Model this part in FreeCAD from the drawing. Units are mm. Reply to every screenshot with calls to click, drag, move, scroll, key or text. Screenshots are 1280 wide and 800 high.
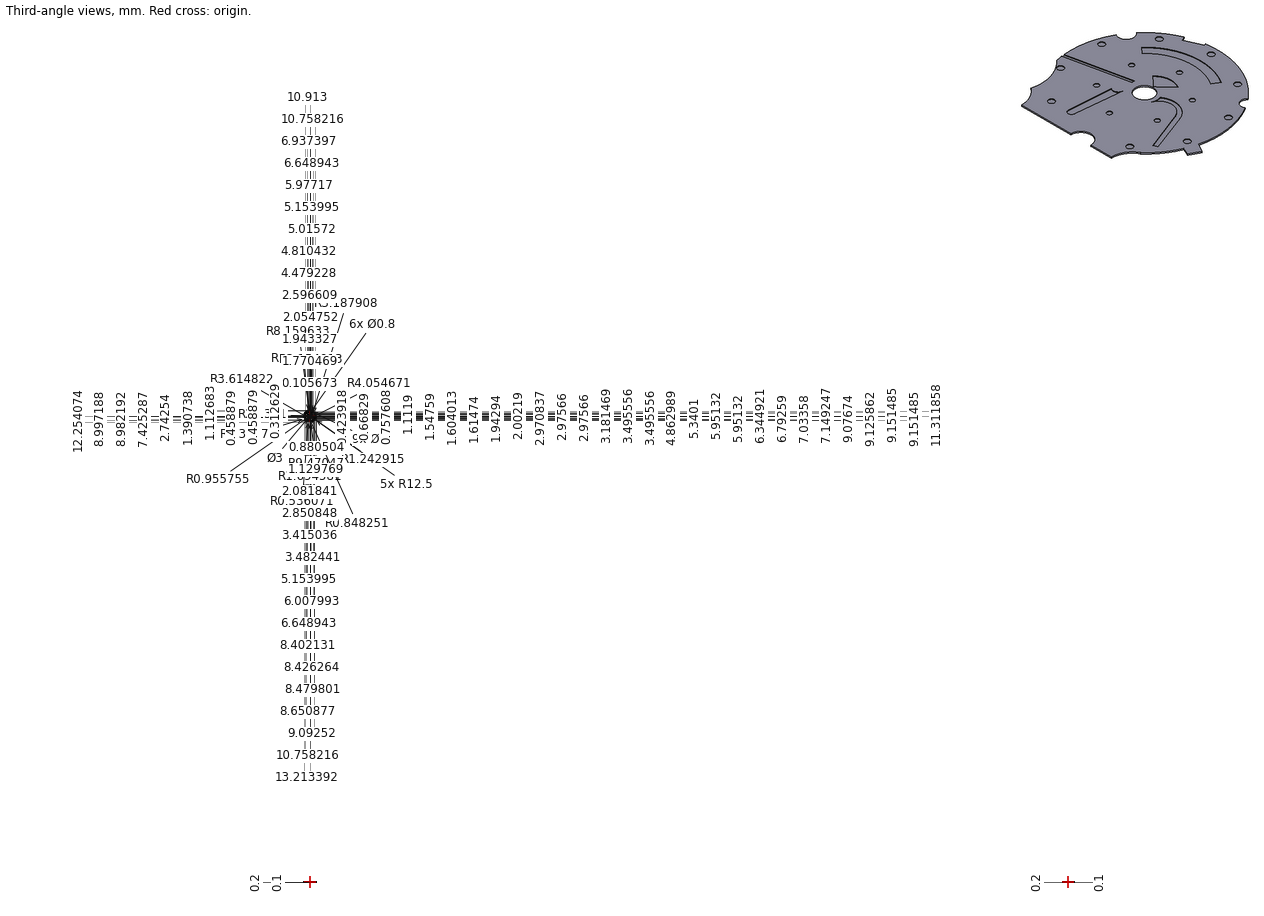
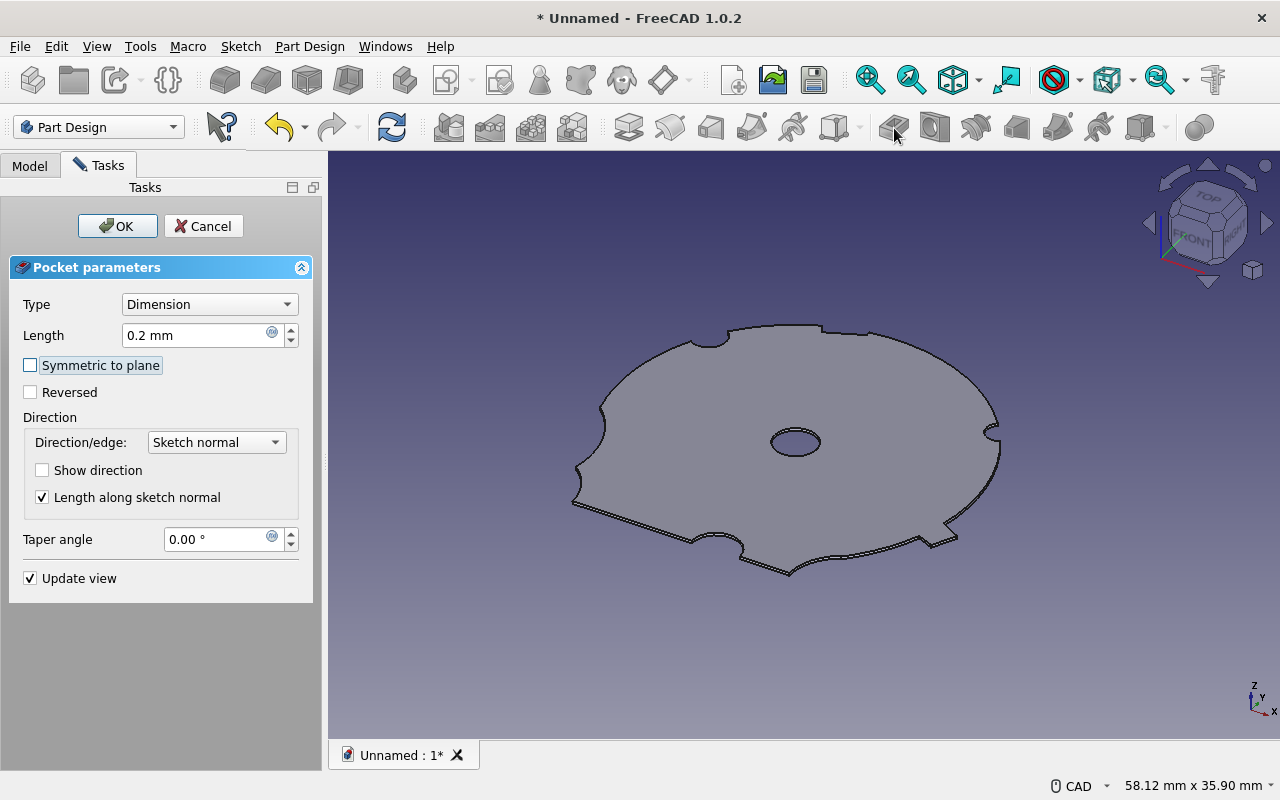
click(118, 226)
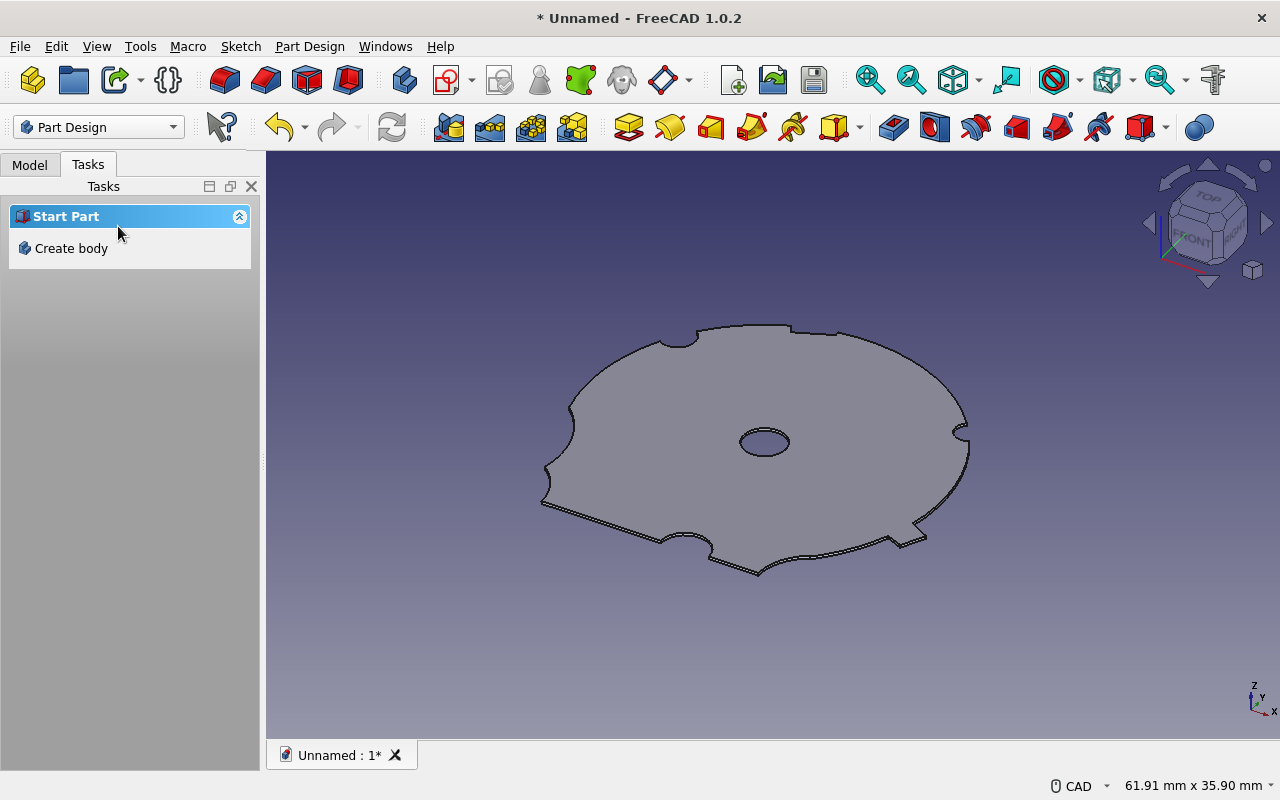
click(668, 408)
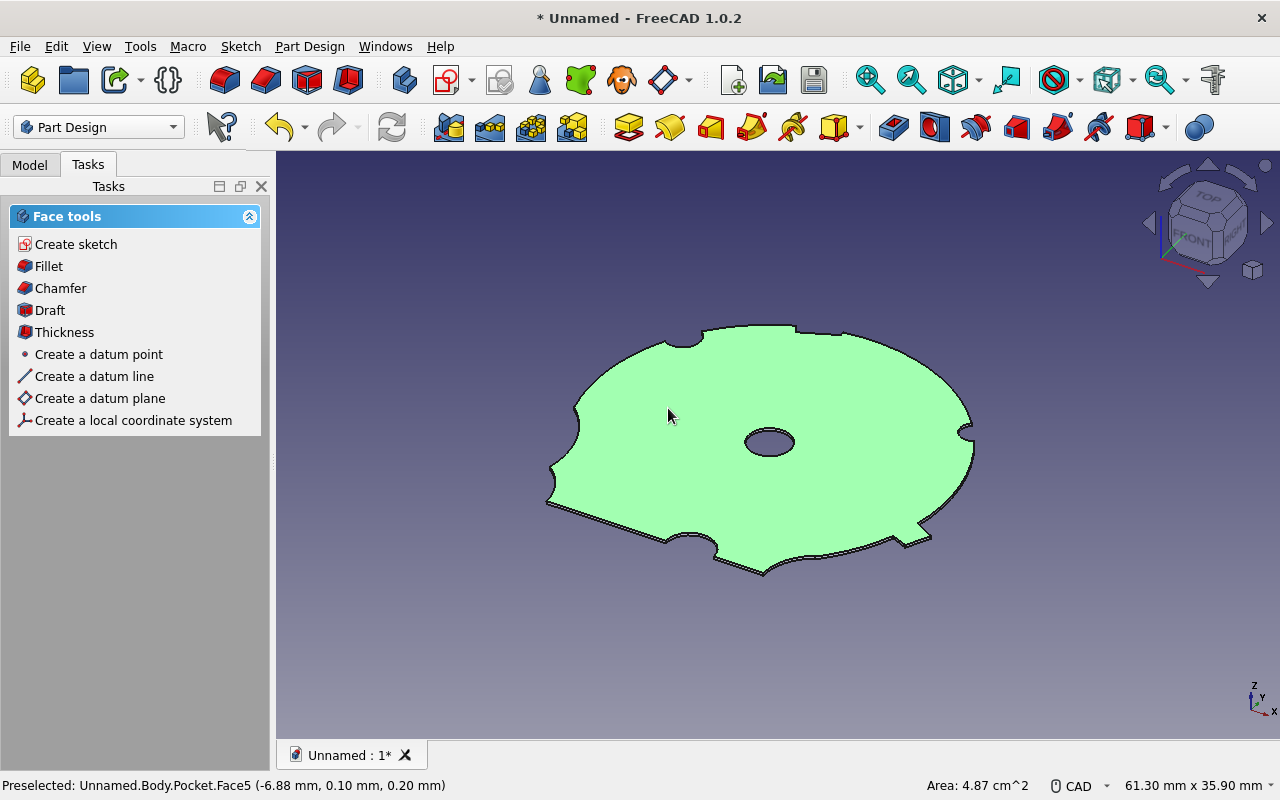
click(446, 80)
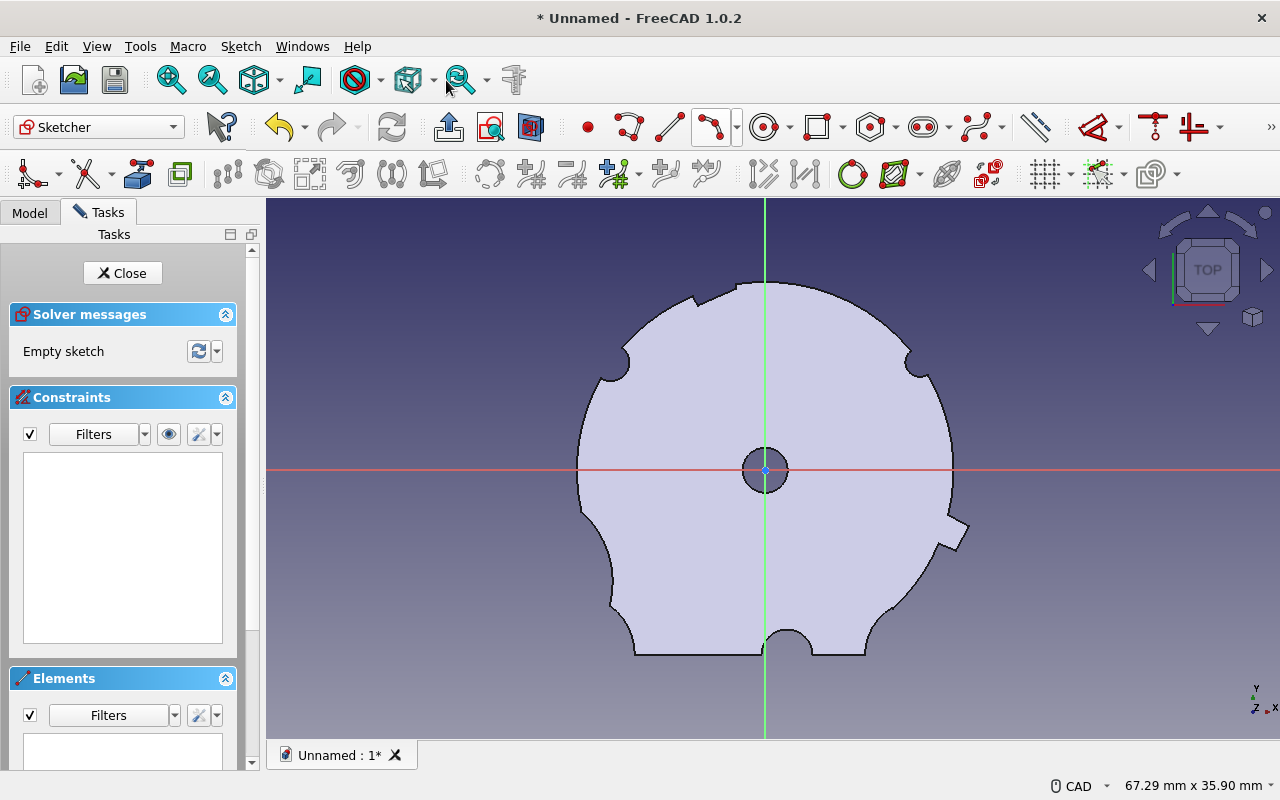
key(g)
key(c)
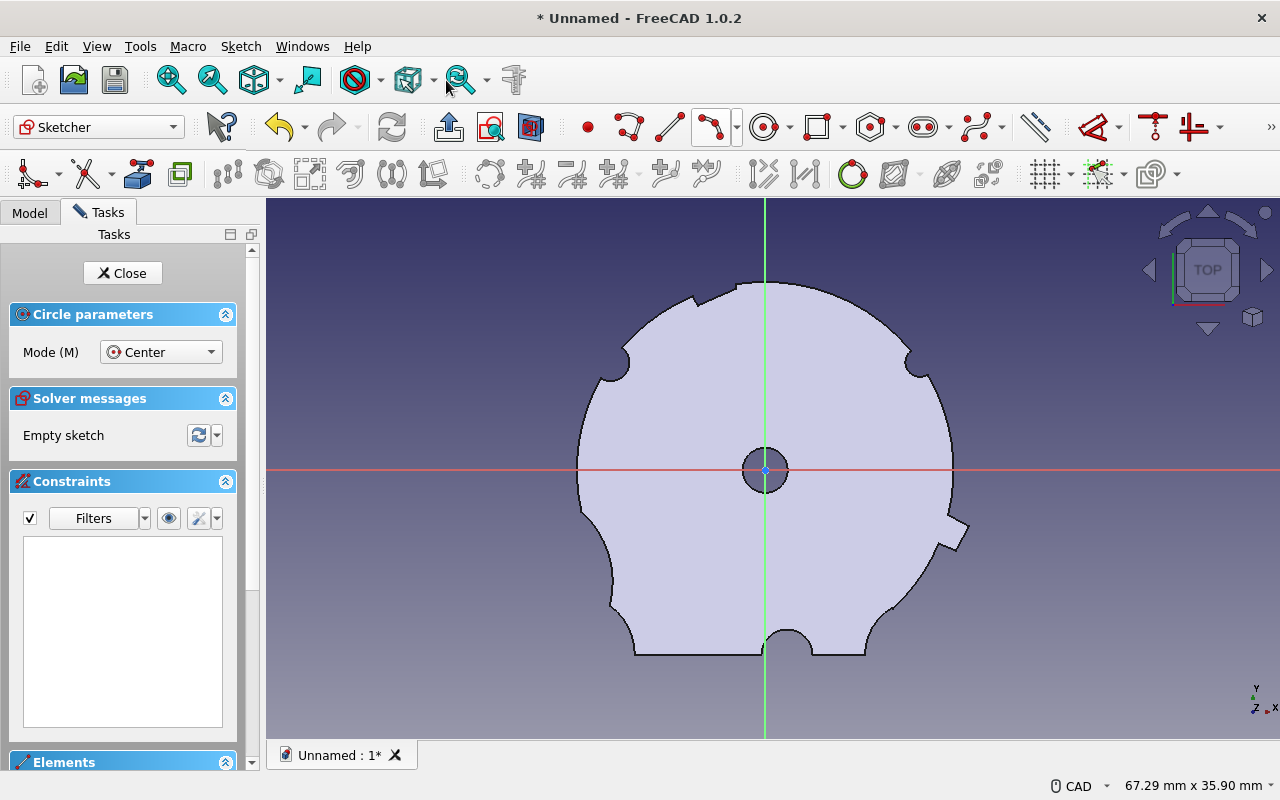
scroll(765, 300, up, 6)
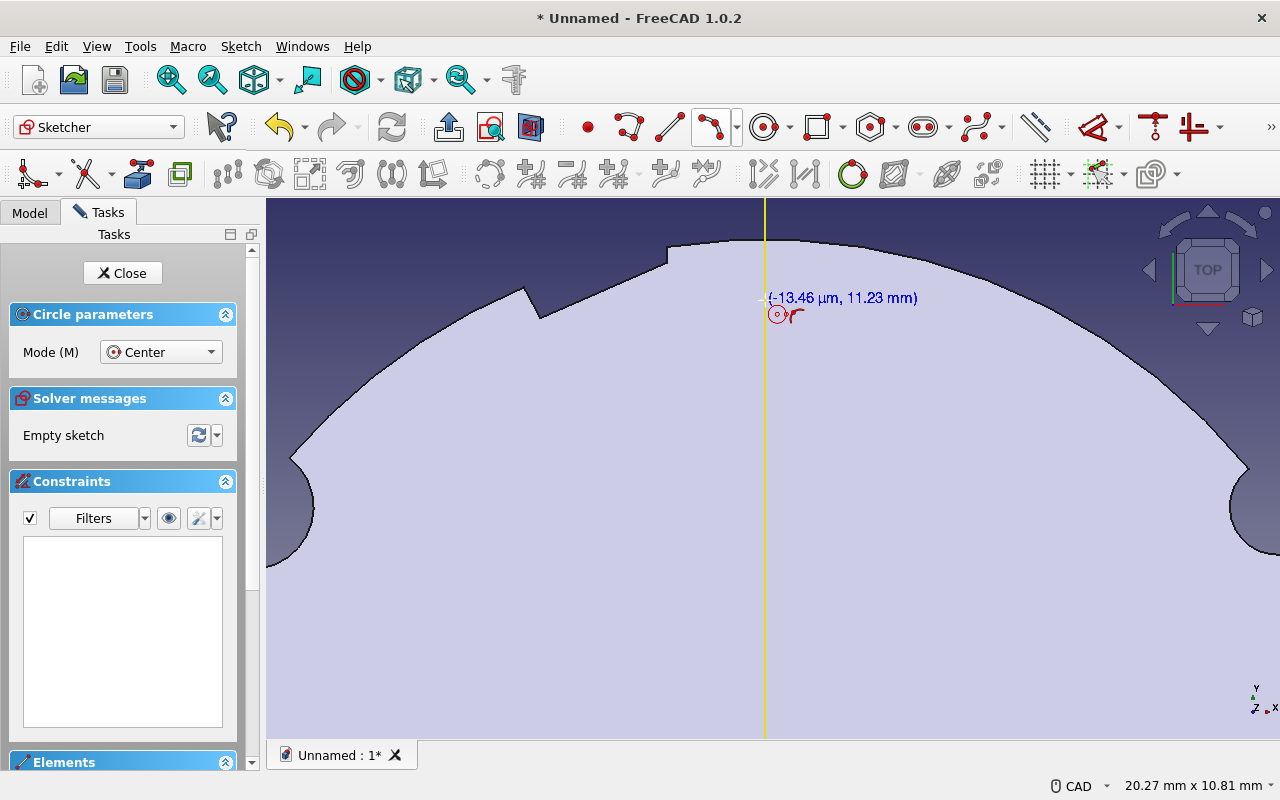
click(765, 299)
click(782, 281)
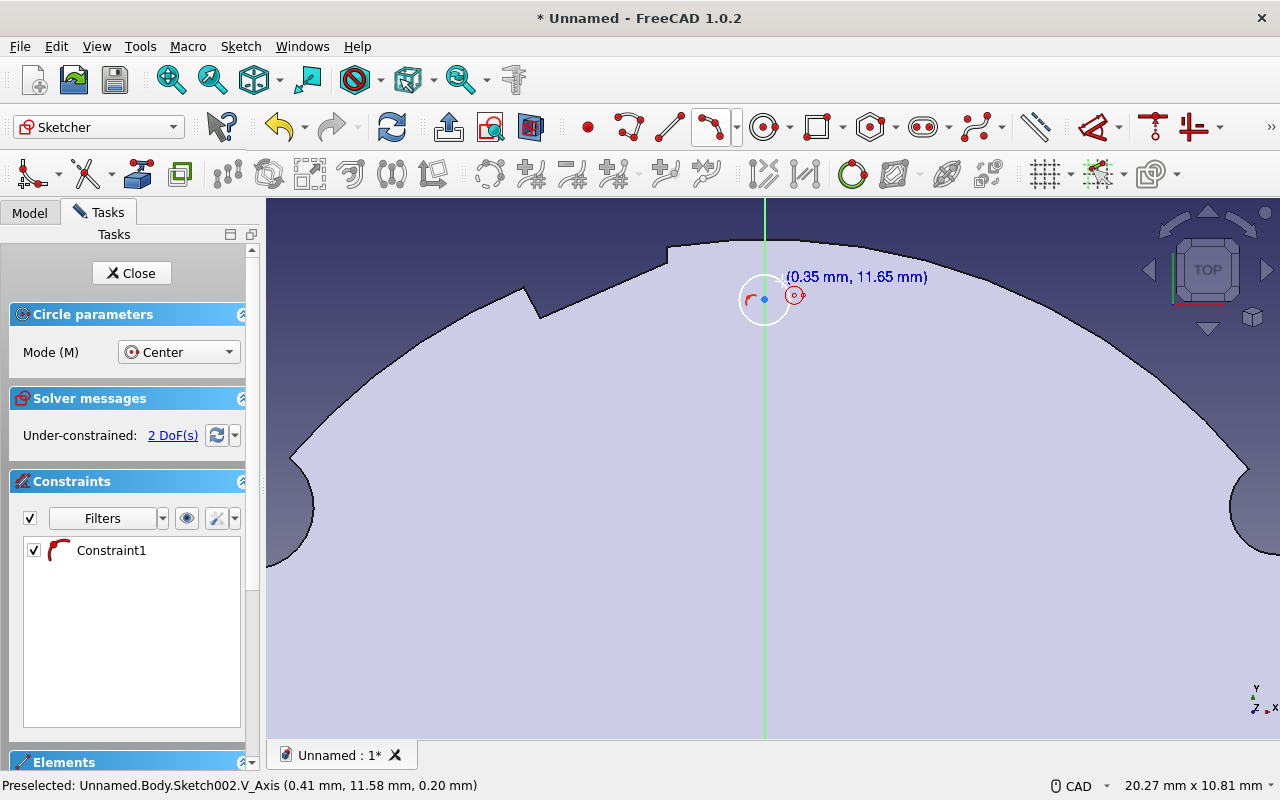
click(1097, 407)
click(1115, 389)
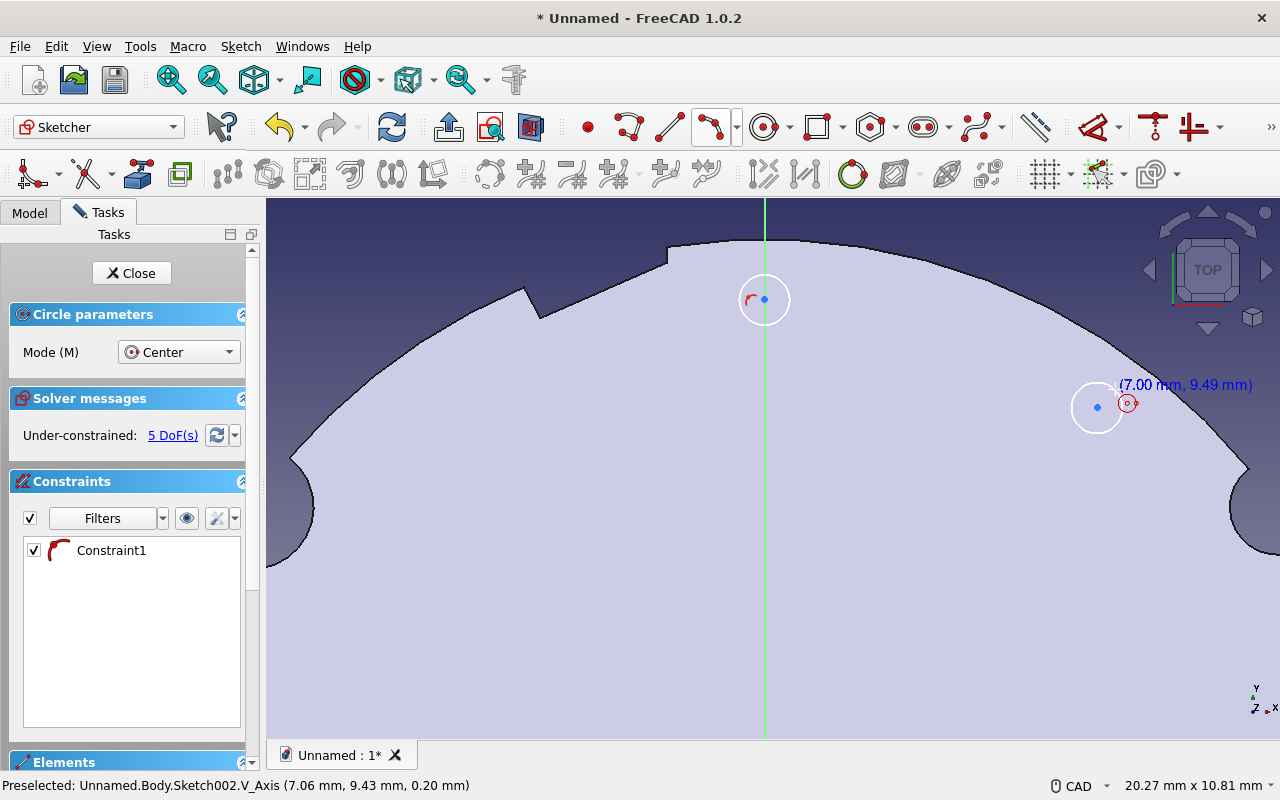
scroll(679, 321, down, 6)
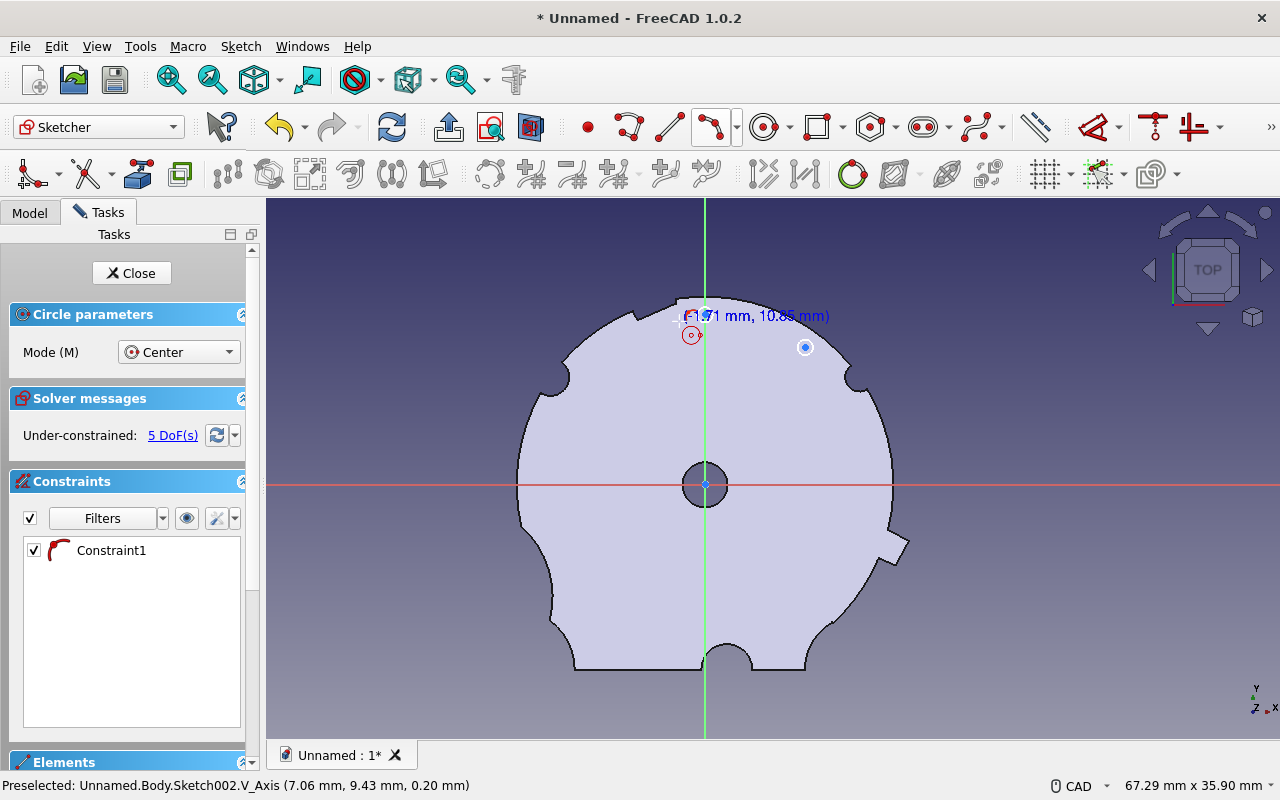
scroll(867, 432, up, 6)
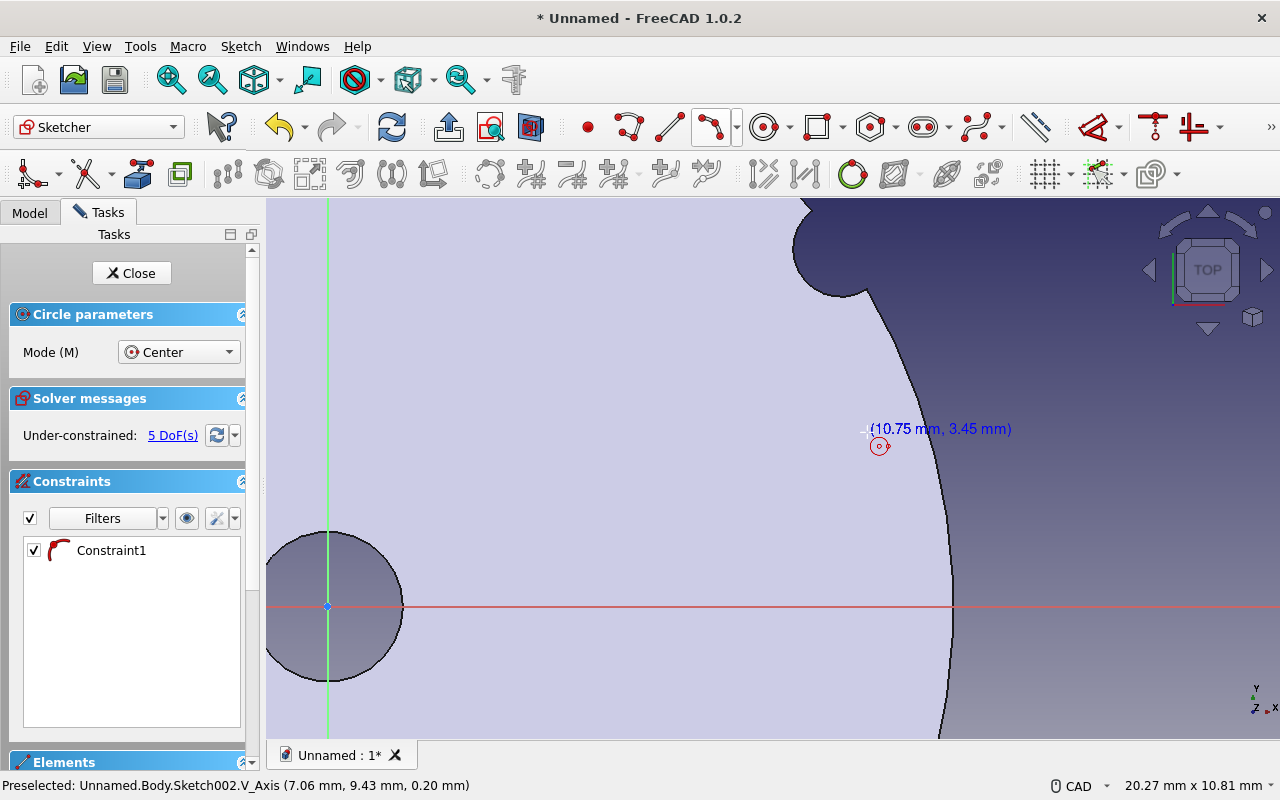
click(866, 432)
click(884, 414)